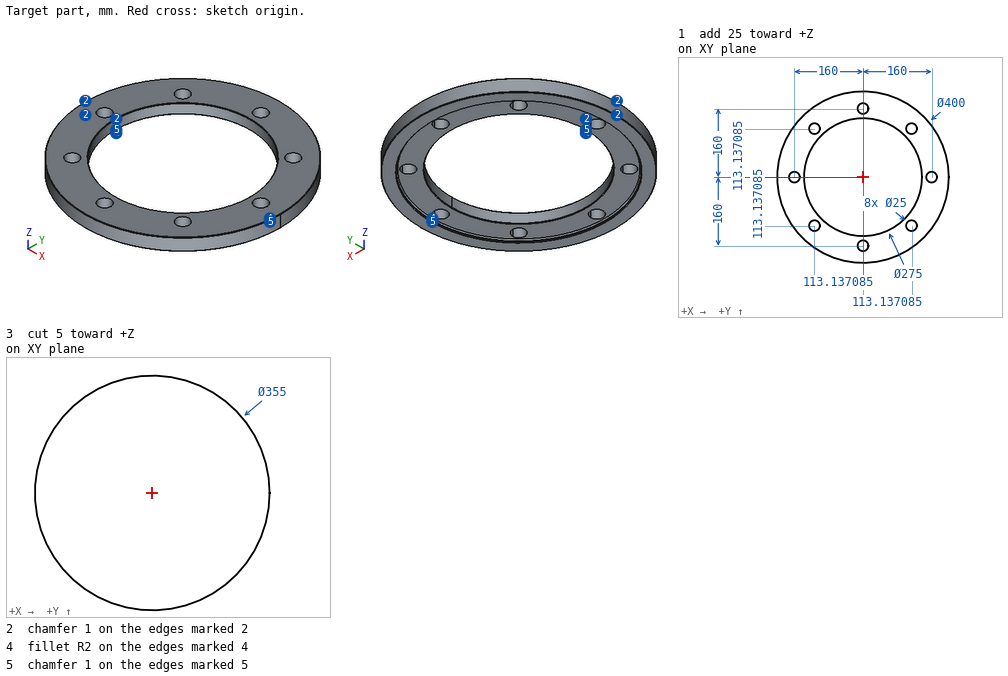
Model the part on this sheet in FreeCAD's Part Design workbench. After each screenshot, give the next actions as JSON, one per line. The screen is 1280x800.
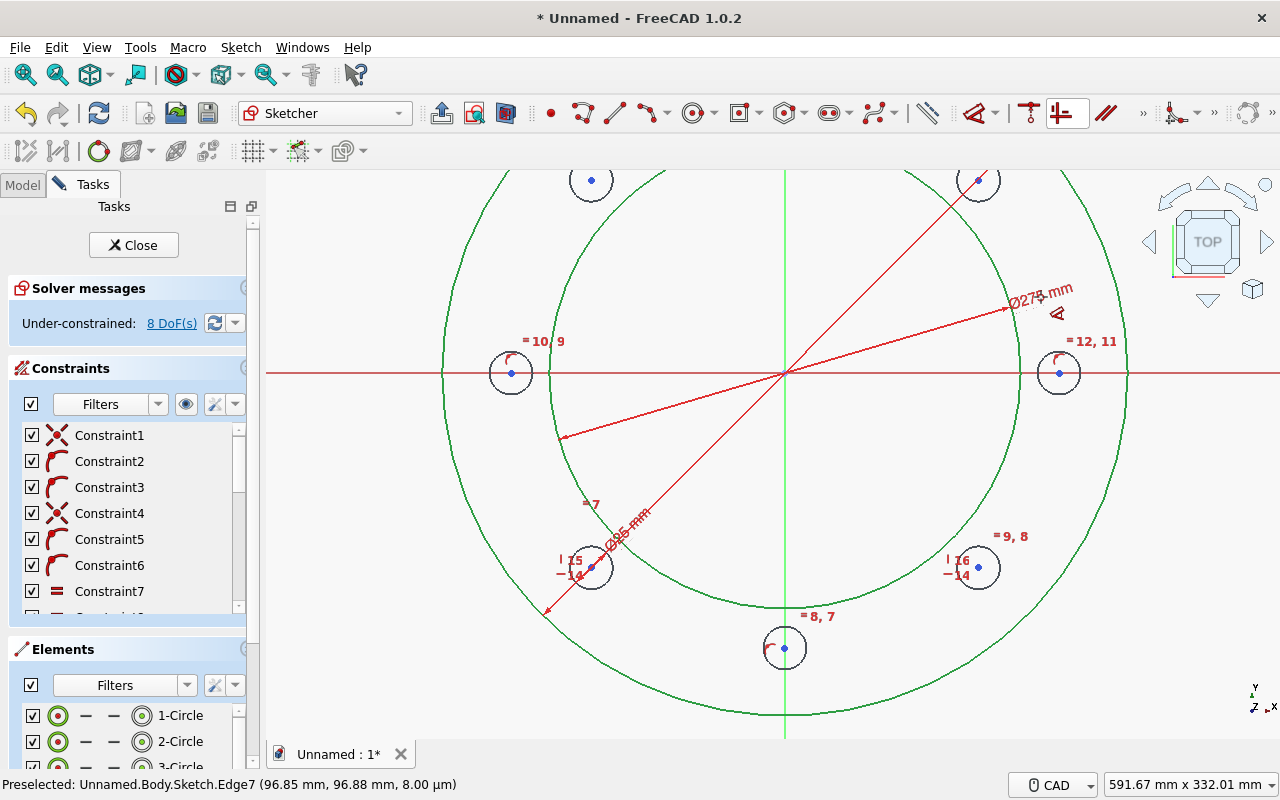
{"action": "left_click", "coordinate": [785, 648]}
{"action": "left_click", "coordinate": [819, 511]}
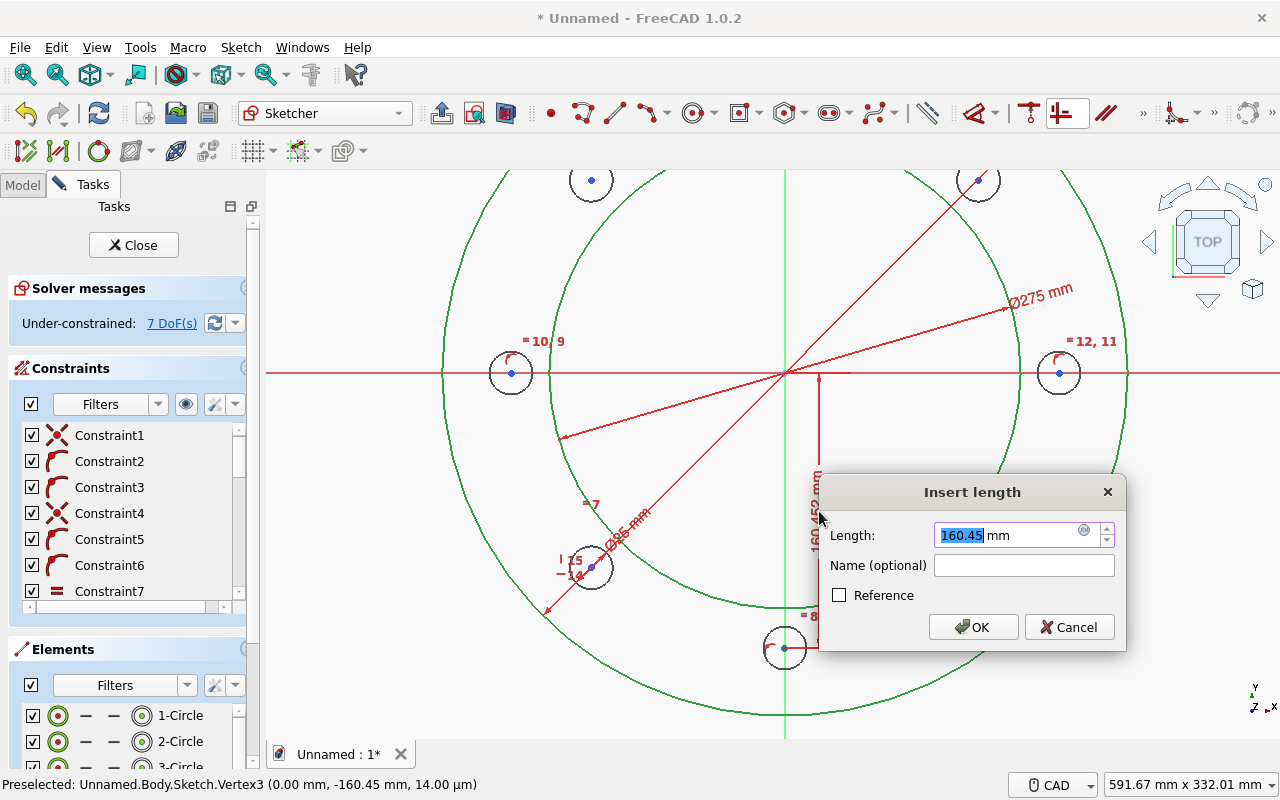
{"action": "type", "text": "160"}
{"action": "key", "text": "Return"}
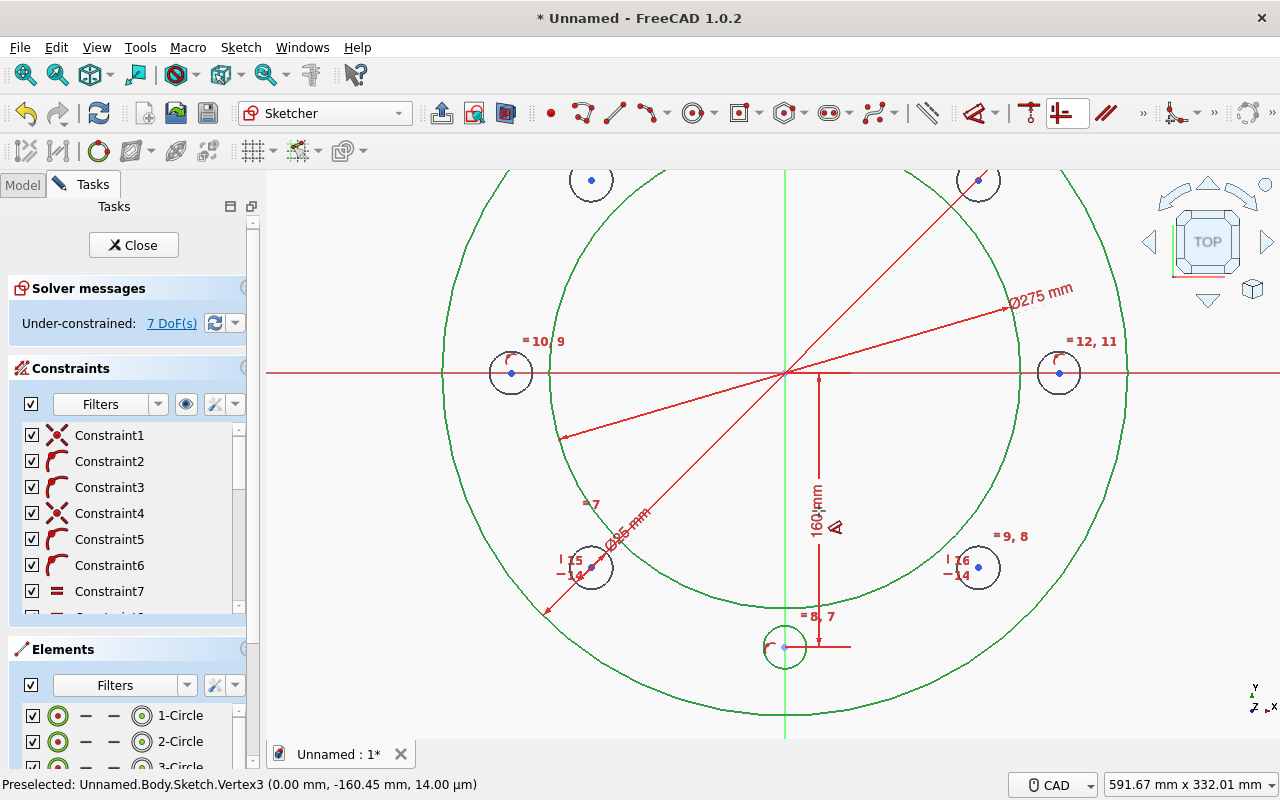
{"action": "left_click", "coordinate": [511, 373]}
{"action": "left_click", "coordinate": [648, 407]}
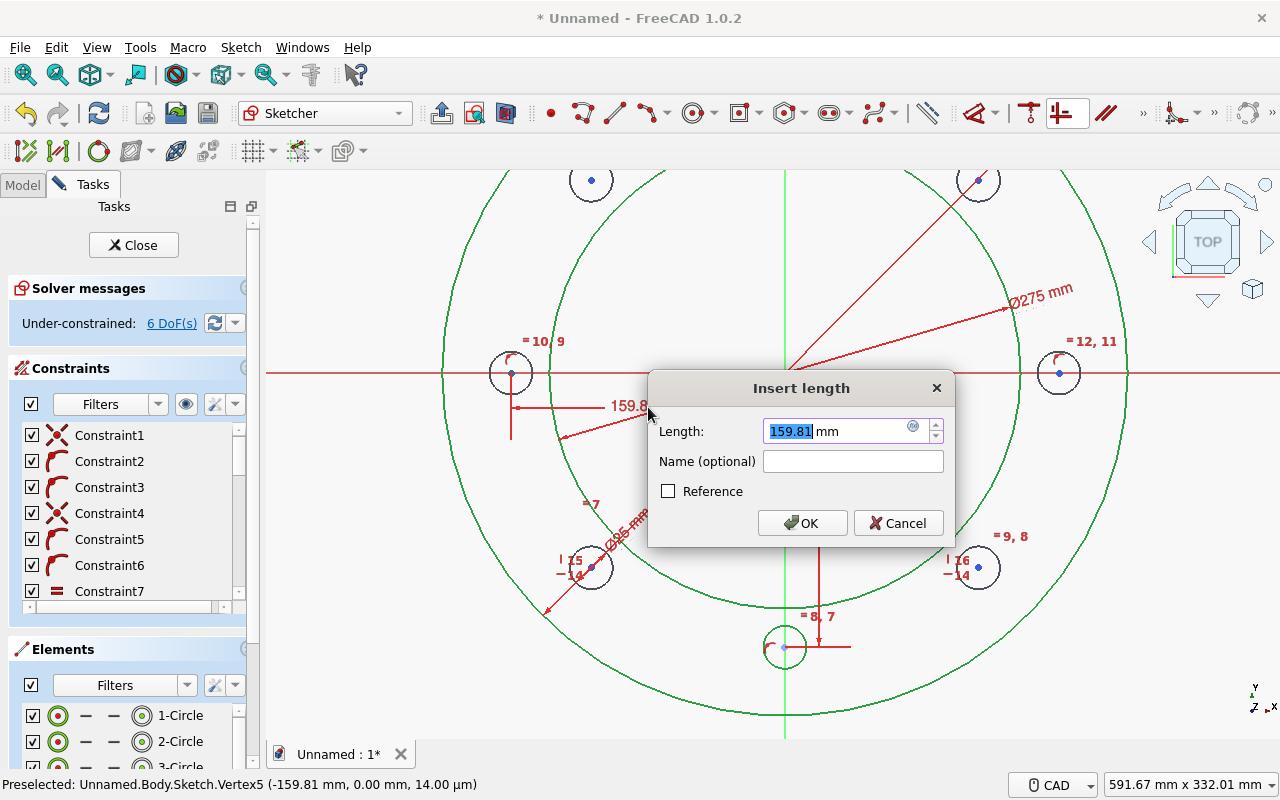
{"action": "type", "text": "160"}
{"action": "key", "text": "Return"}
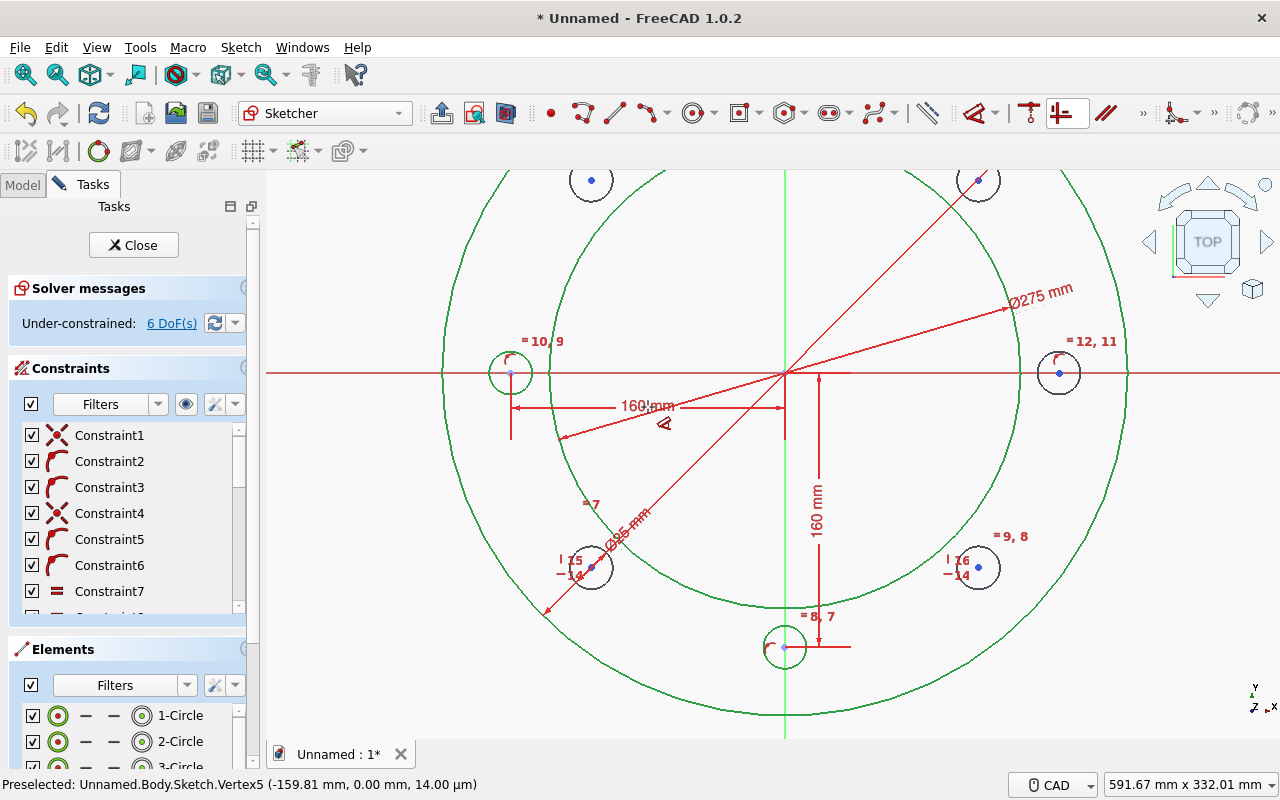
{"action": "left_click", "coordinate": [1059, 373]}
{"action": "left_click", "coordinate": [922, 407]}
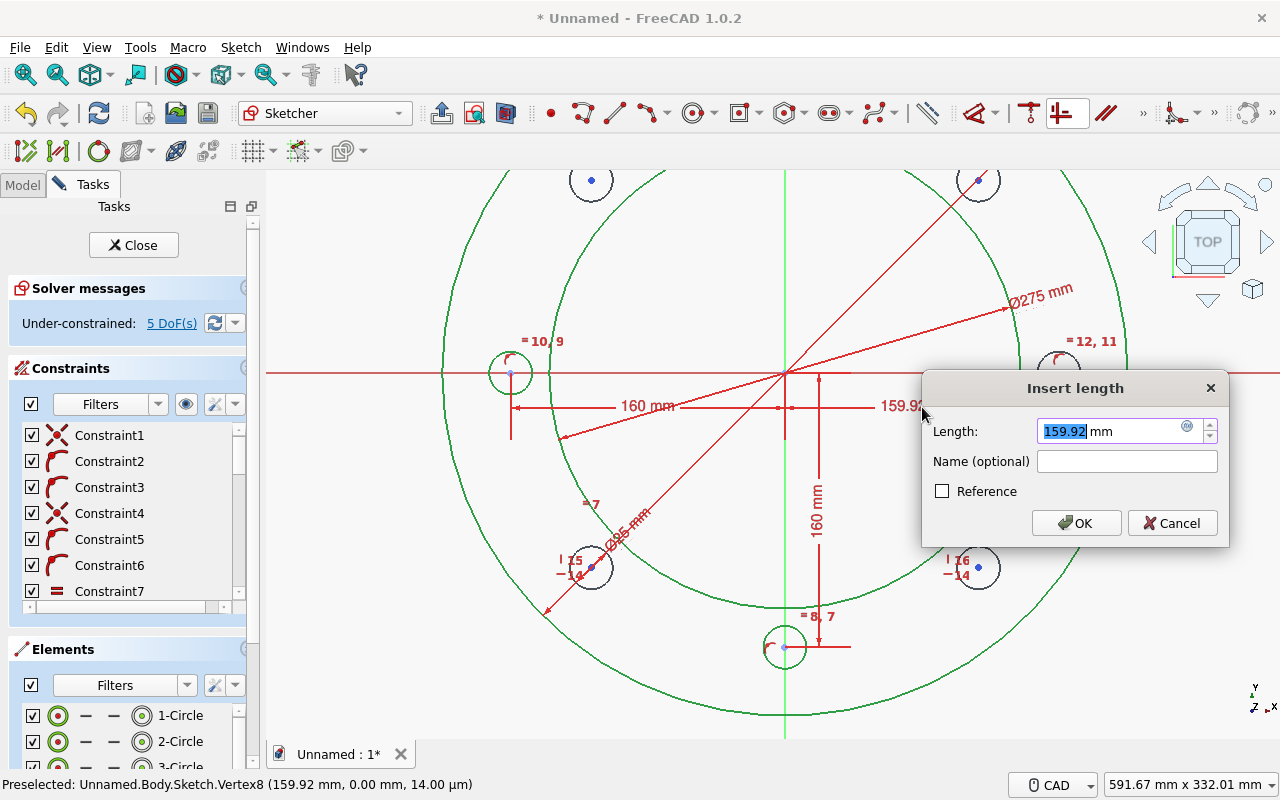
{"action": "type", "text": "160"}
{"action": "key", "text": "Return"}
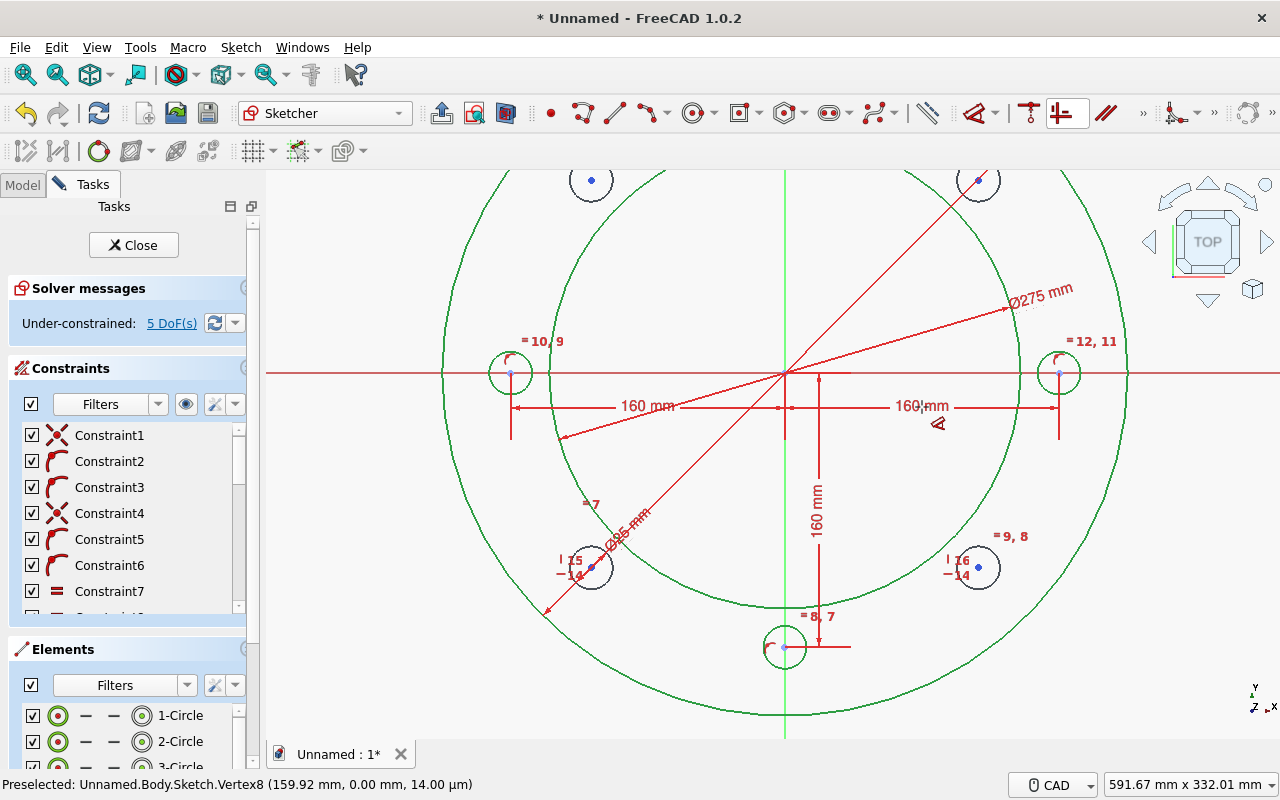
{"action": "scroll", "coordinate": [607, 554], "scroll_direction": "down", "scroll_amount": 3}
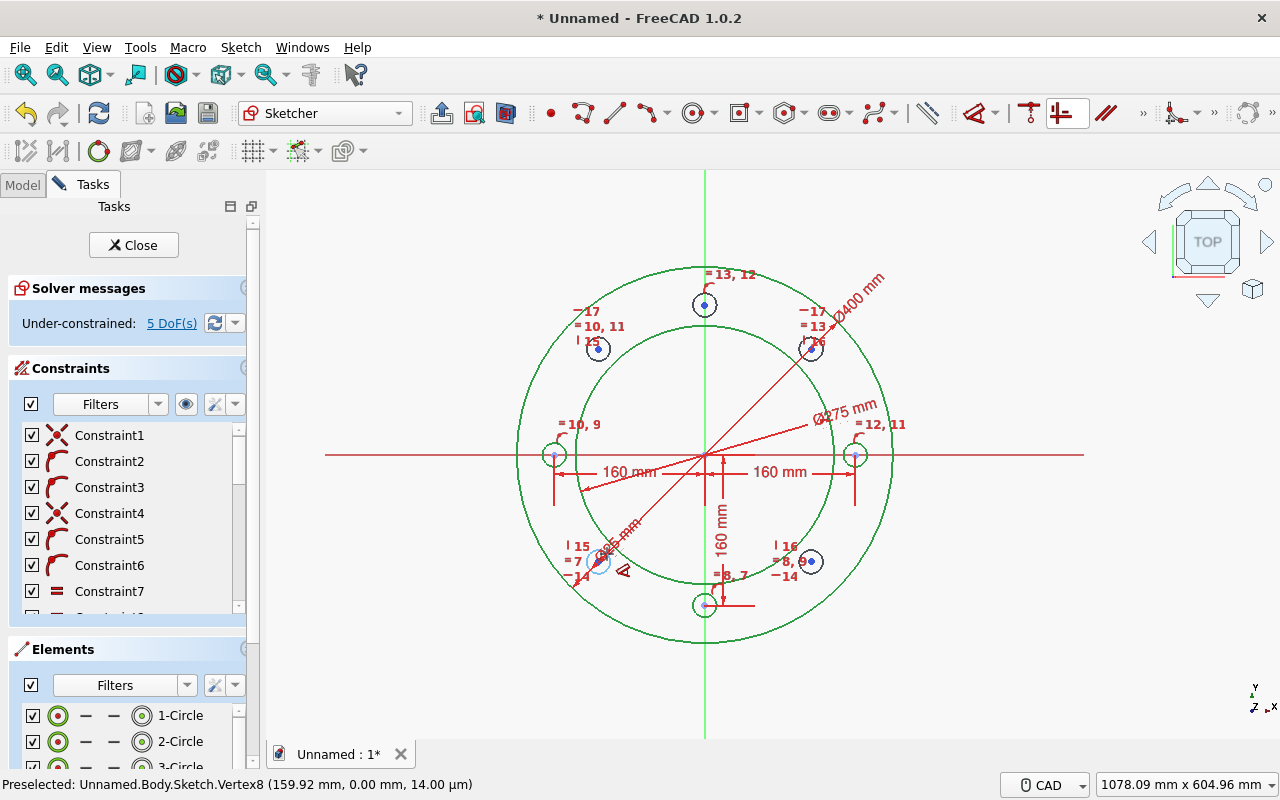
{"action": "left_click", "coordinate": [705, 305]}
{"action": "left_click", "coordinate": [739, 380]}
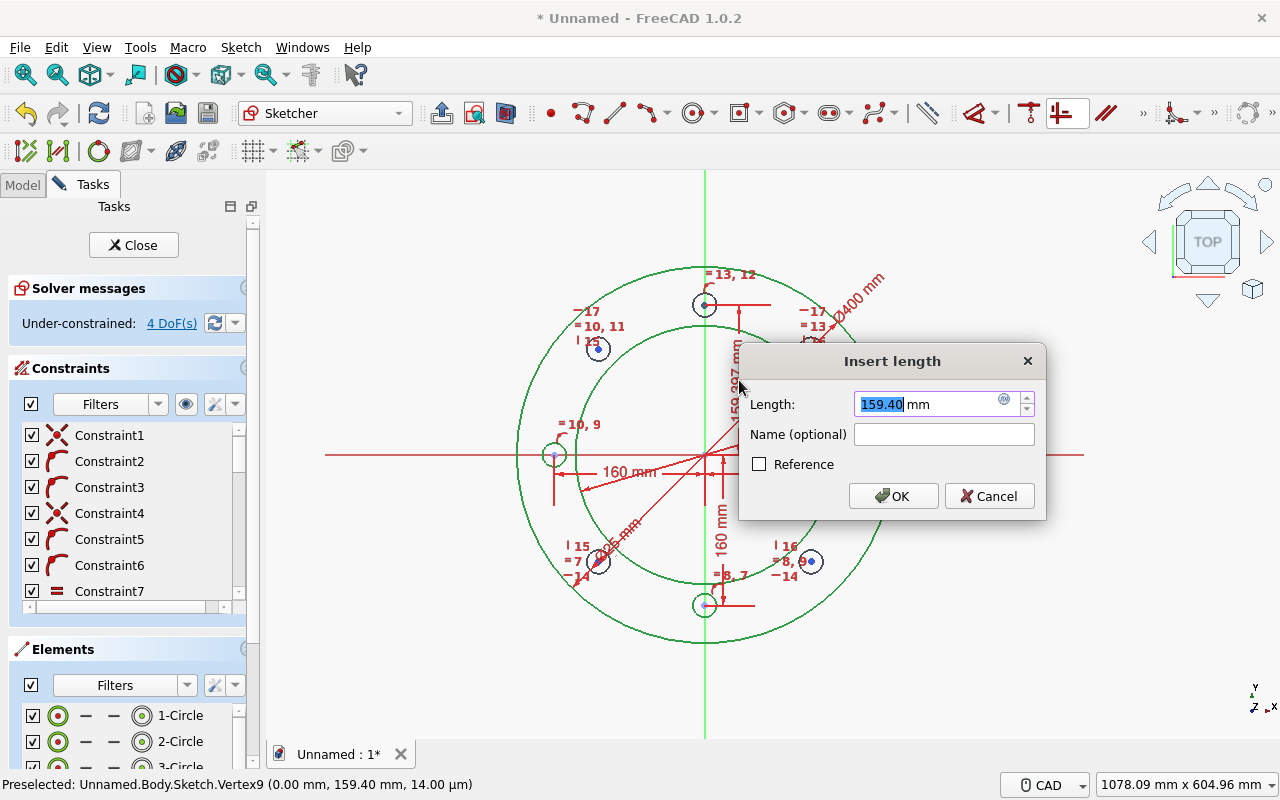
{"action": "type", "text": "160"}
{"action": "key", "text": "Return"}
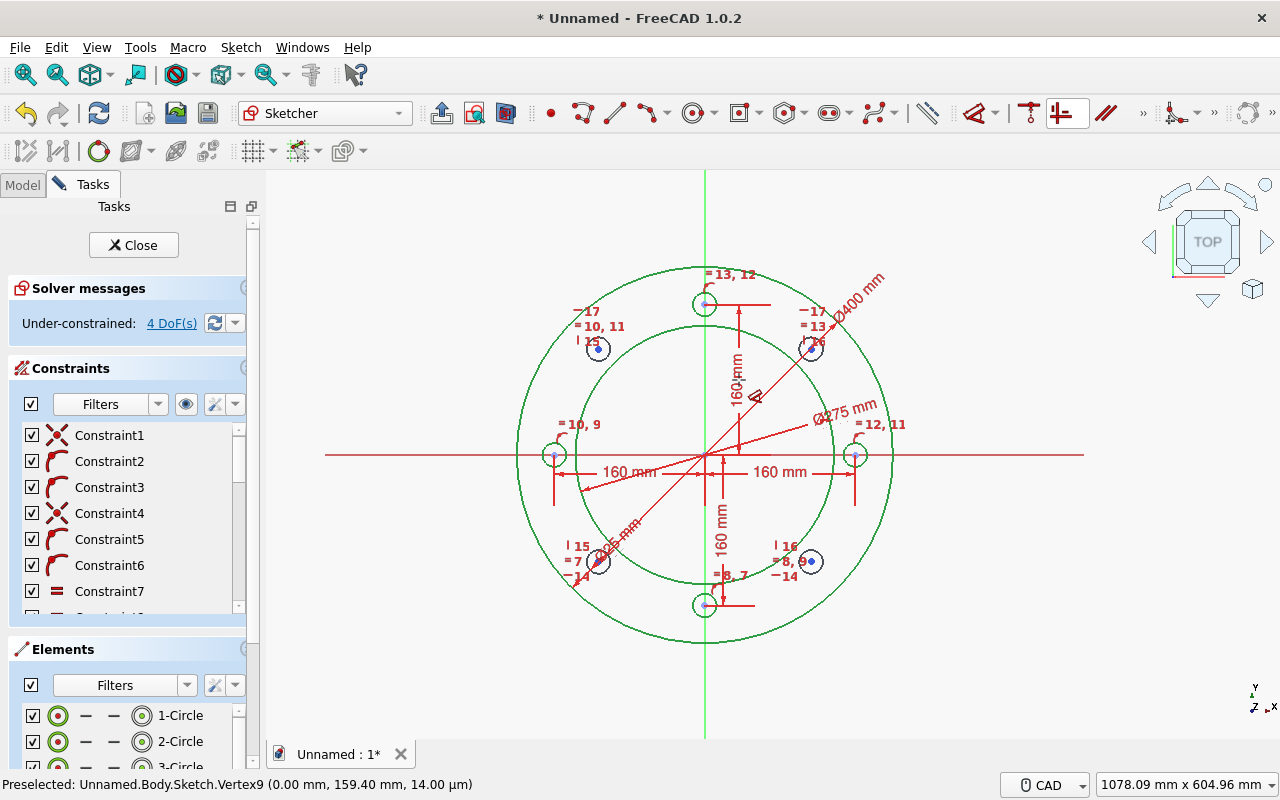
{"action": "left_click", "coordinate": [599, 562]}
{"action": "left_click", "coordinate": [652, 596]}